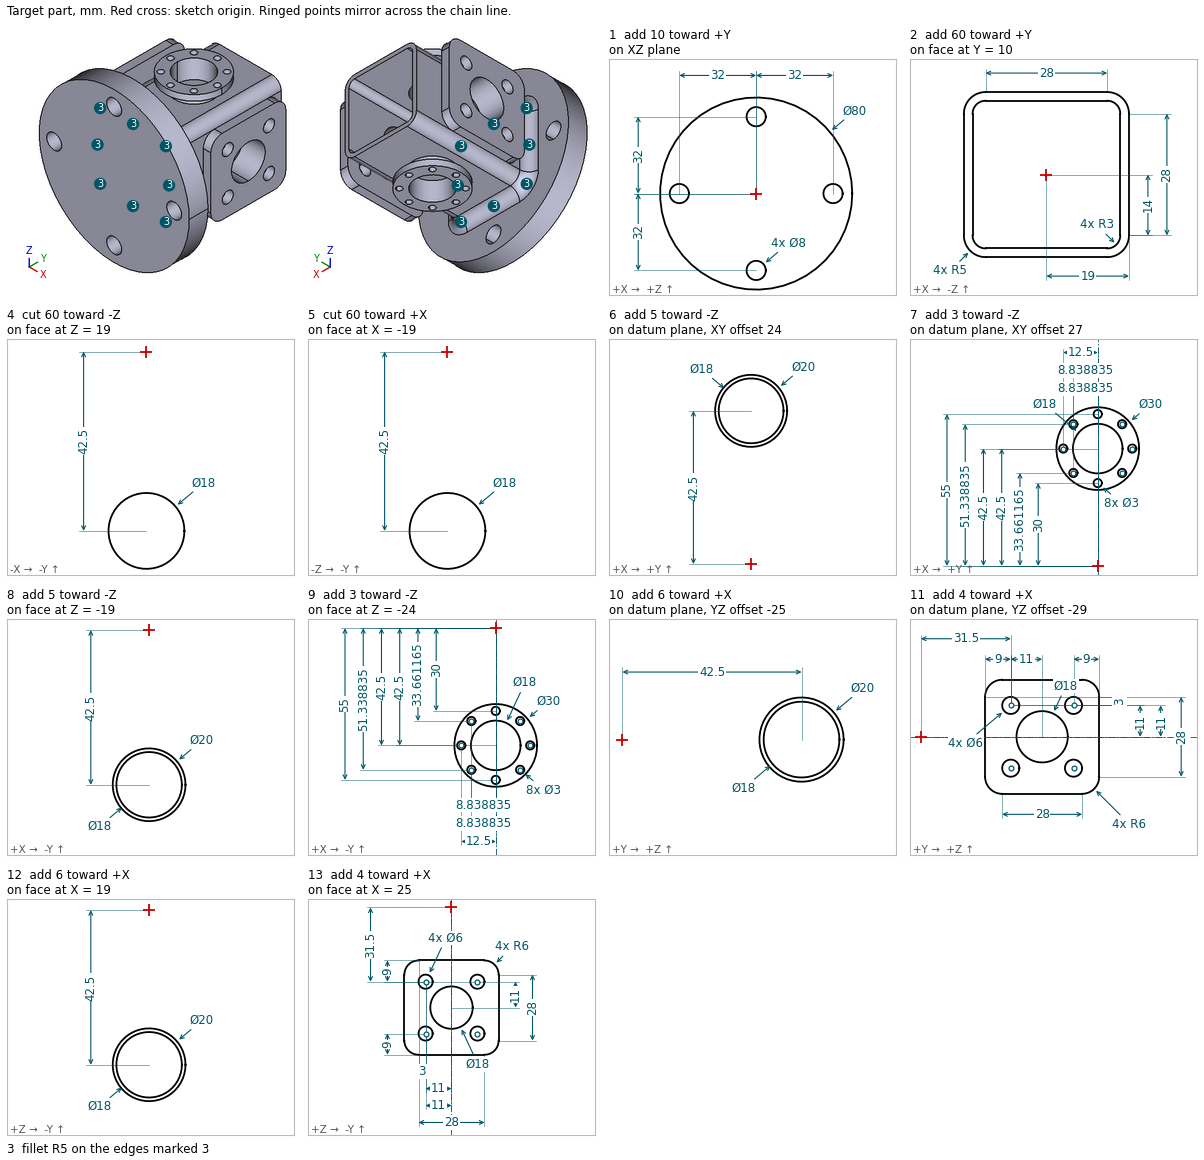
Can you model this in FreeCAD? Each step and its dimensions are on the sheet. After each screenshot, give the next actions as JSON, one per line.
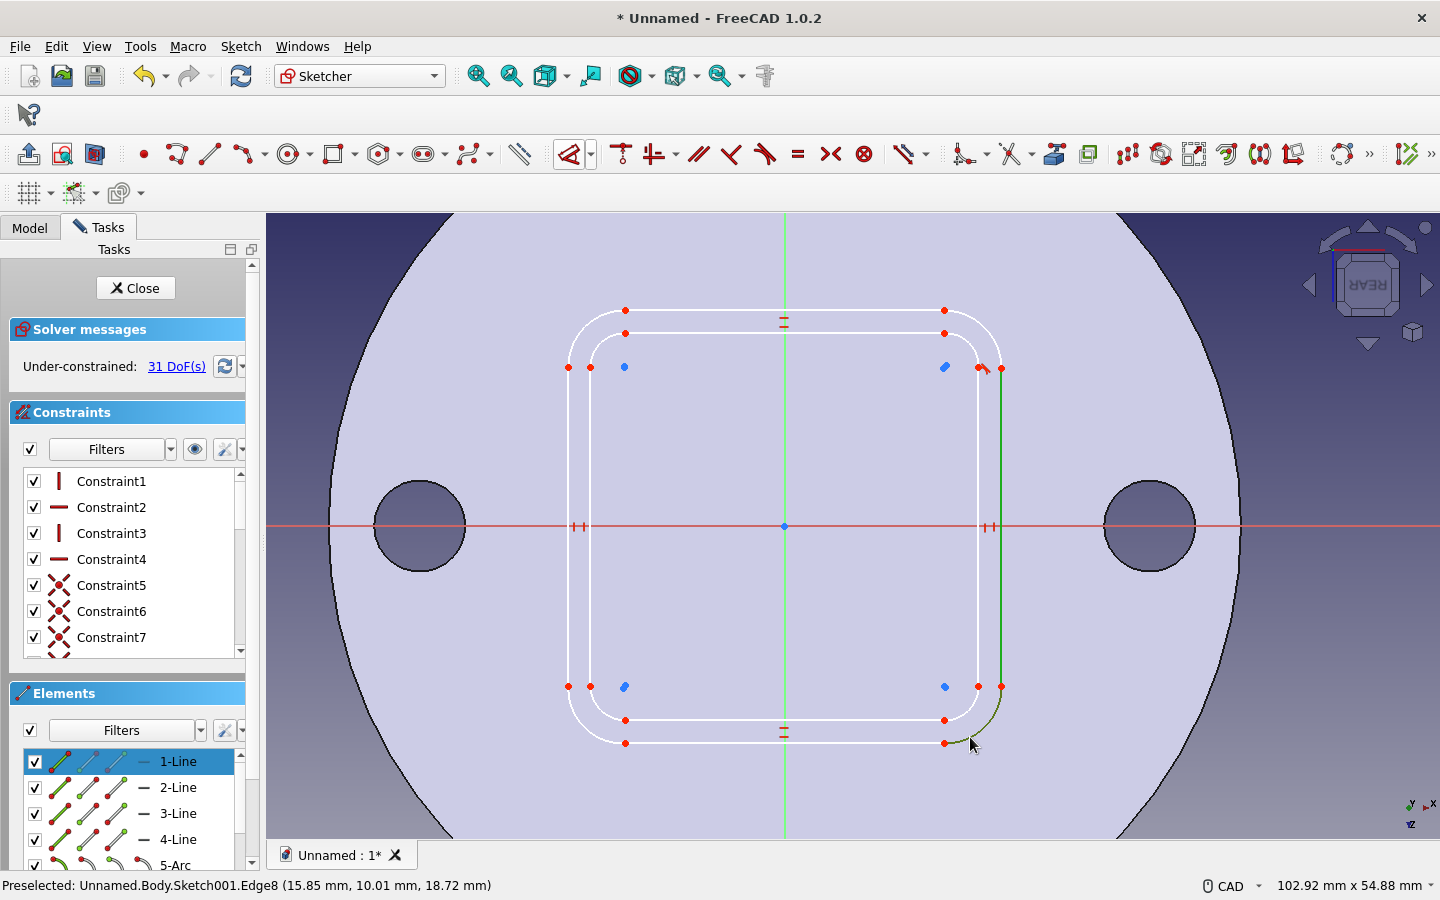
{"action": "key", "text": "t"}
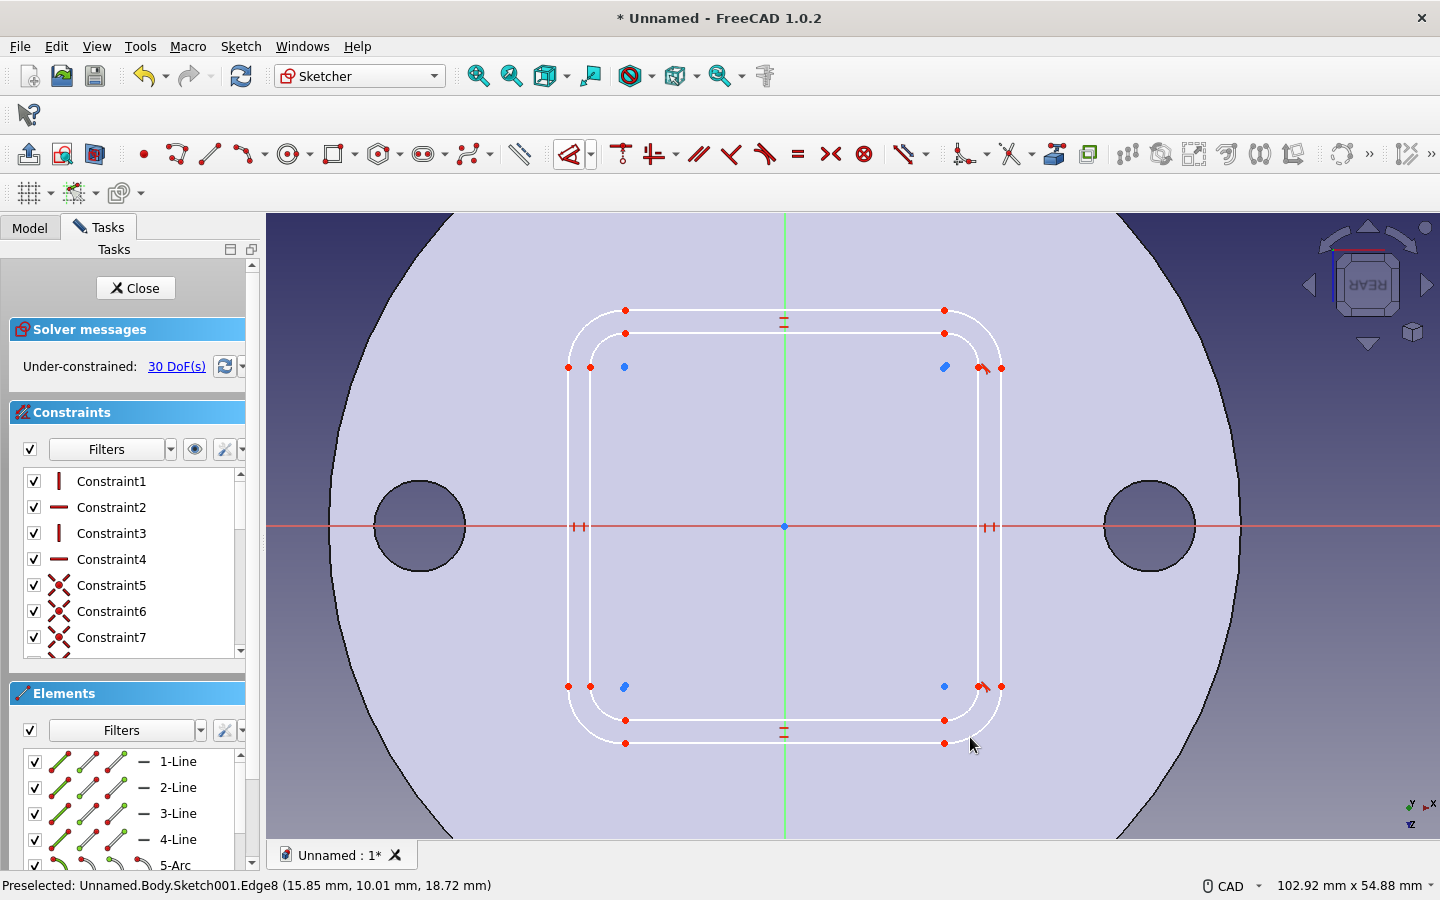
{"action": "left_click", "coordinate": [849, 310]}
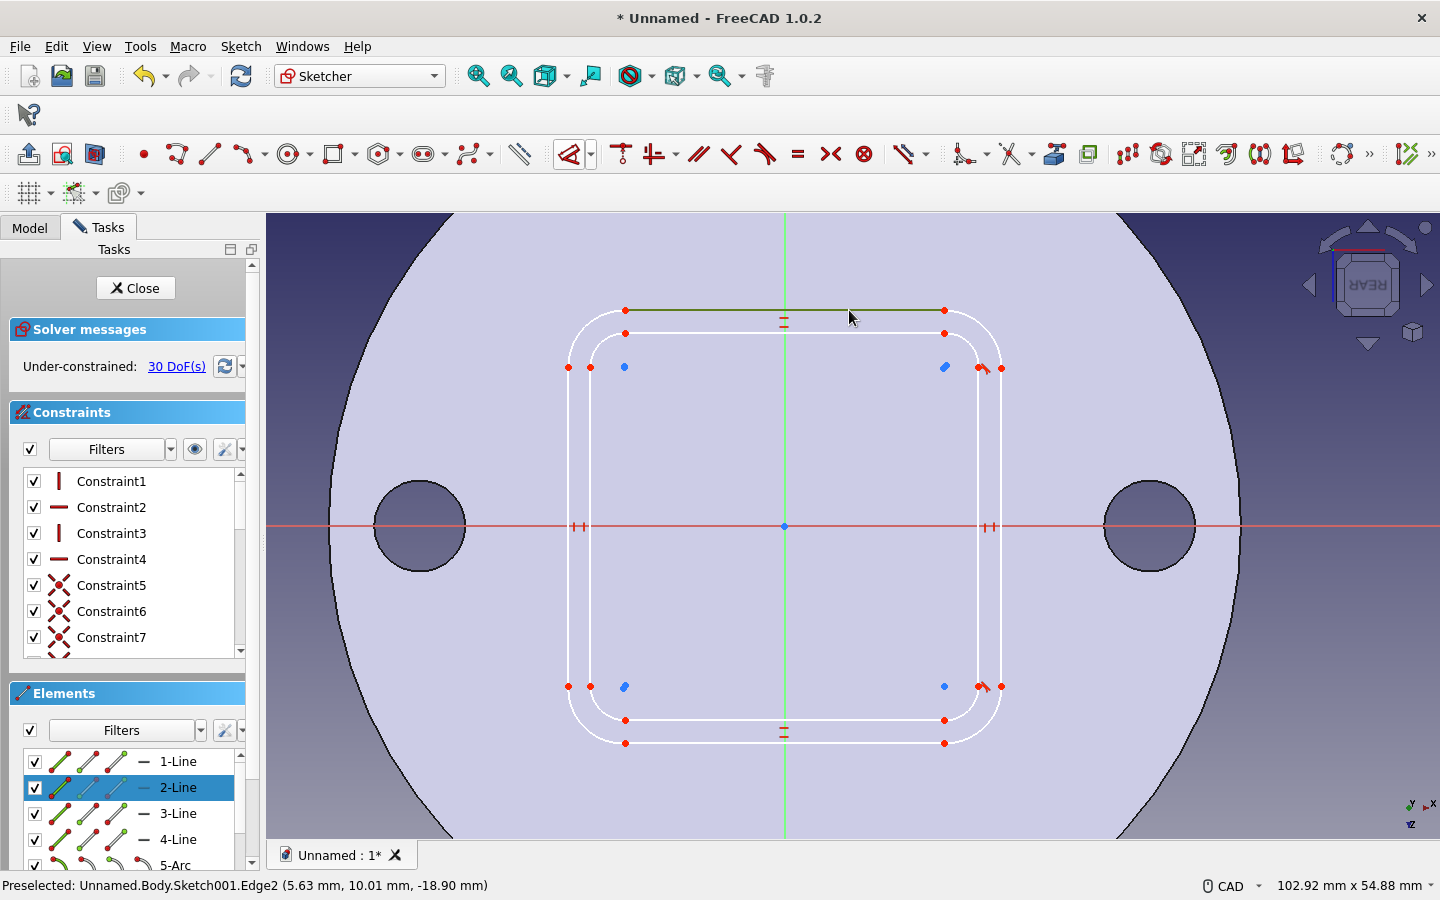
{"action": "left_click", "coordinate": [995, 342]}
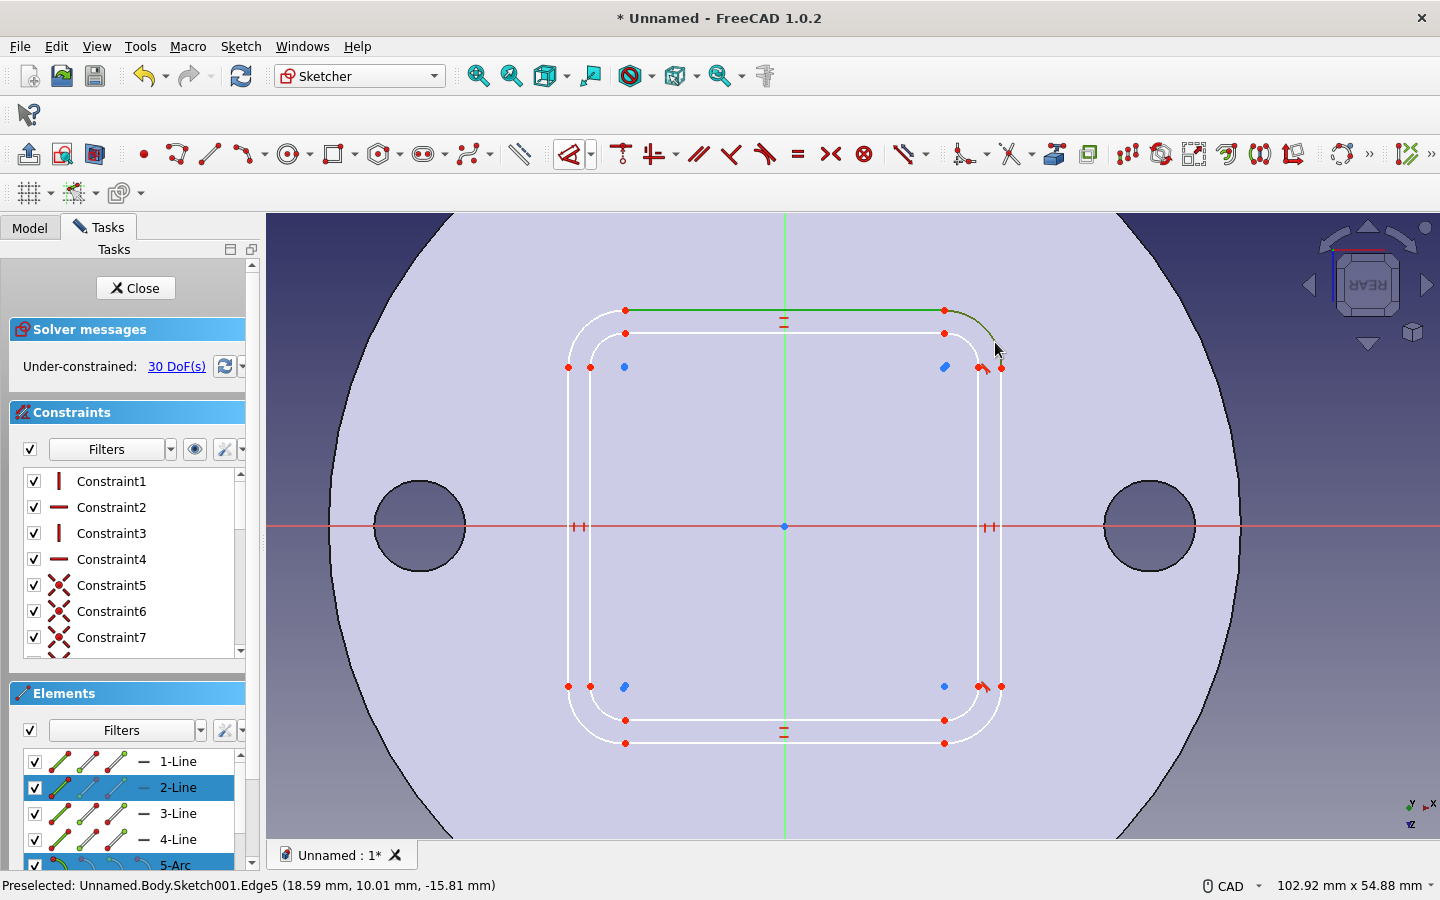
{"action": "key", "text": "t"}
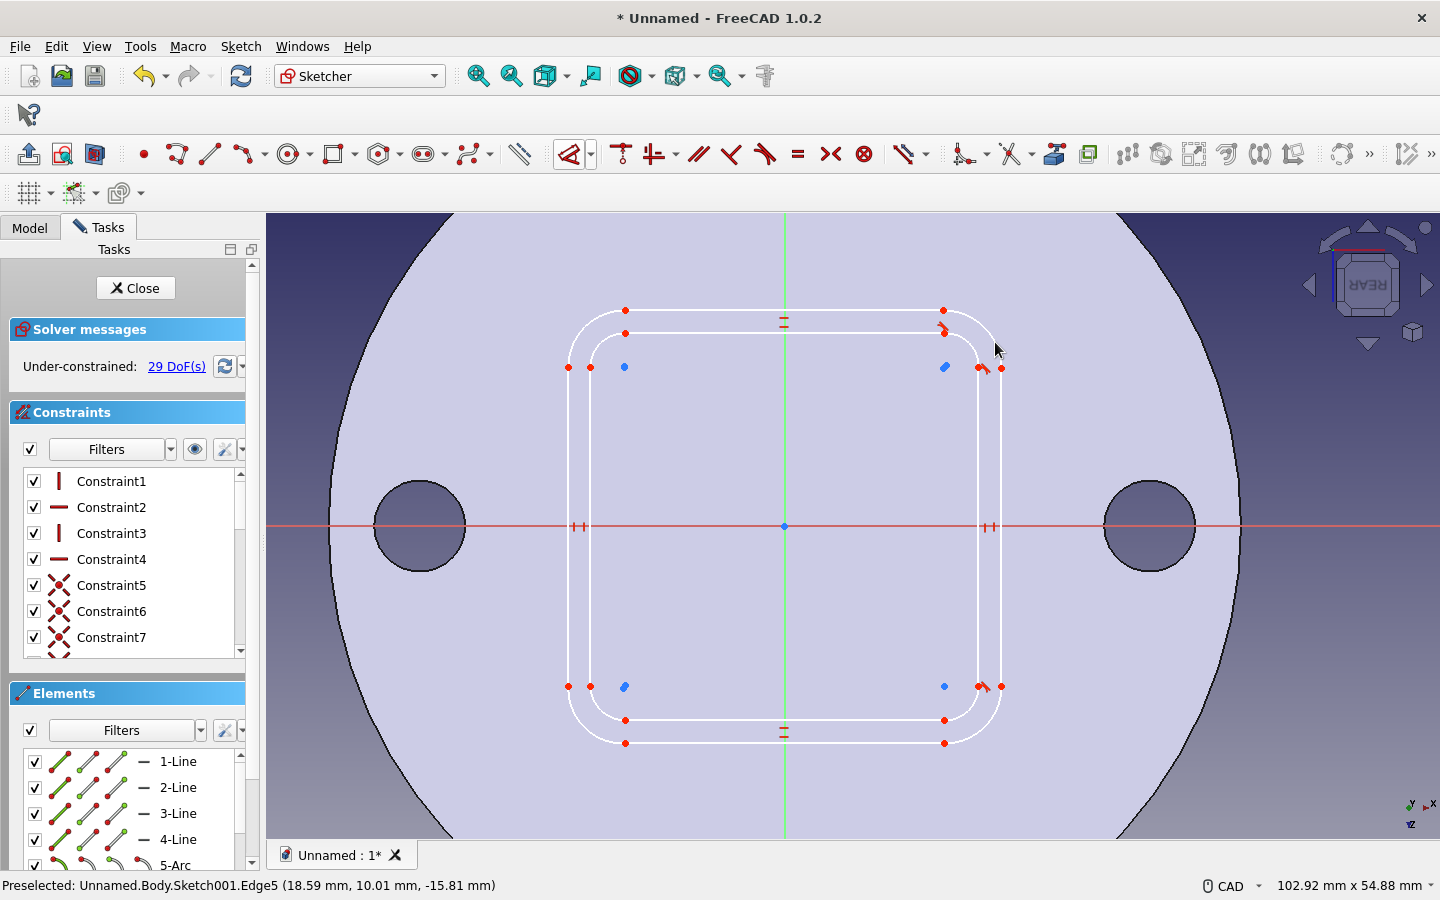
{"action": "left_click", "coordinate": [848, 310]}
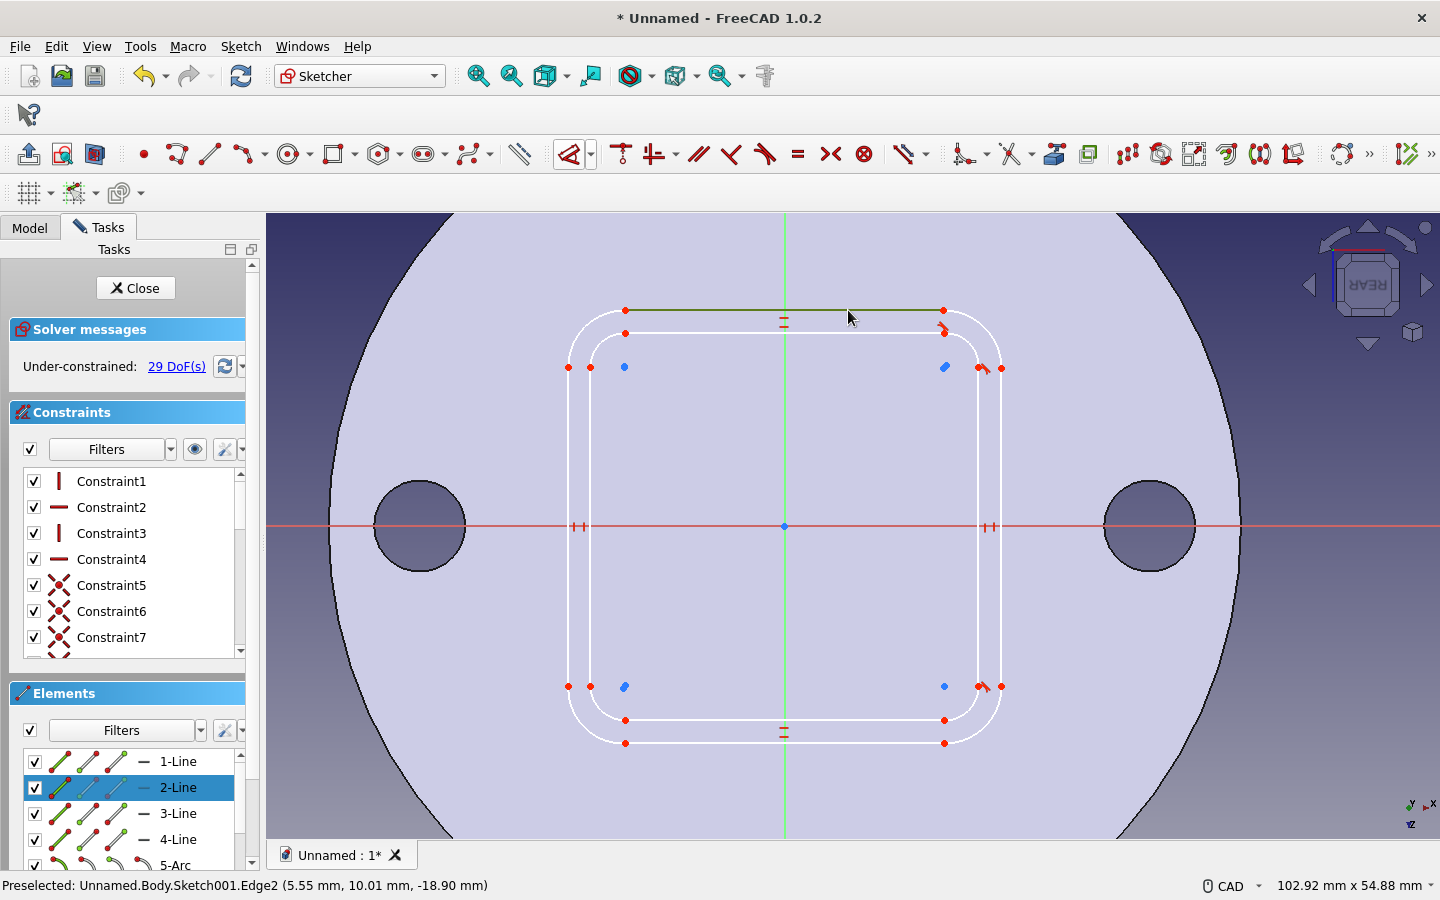
{"action": "left_click", "coordinate": [599, 316]}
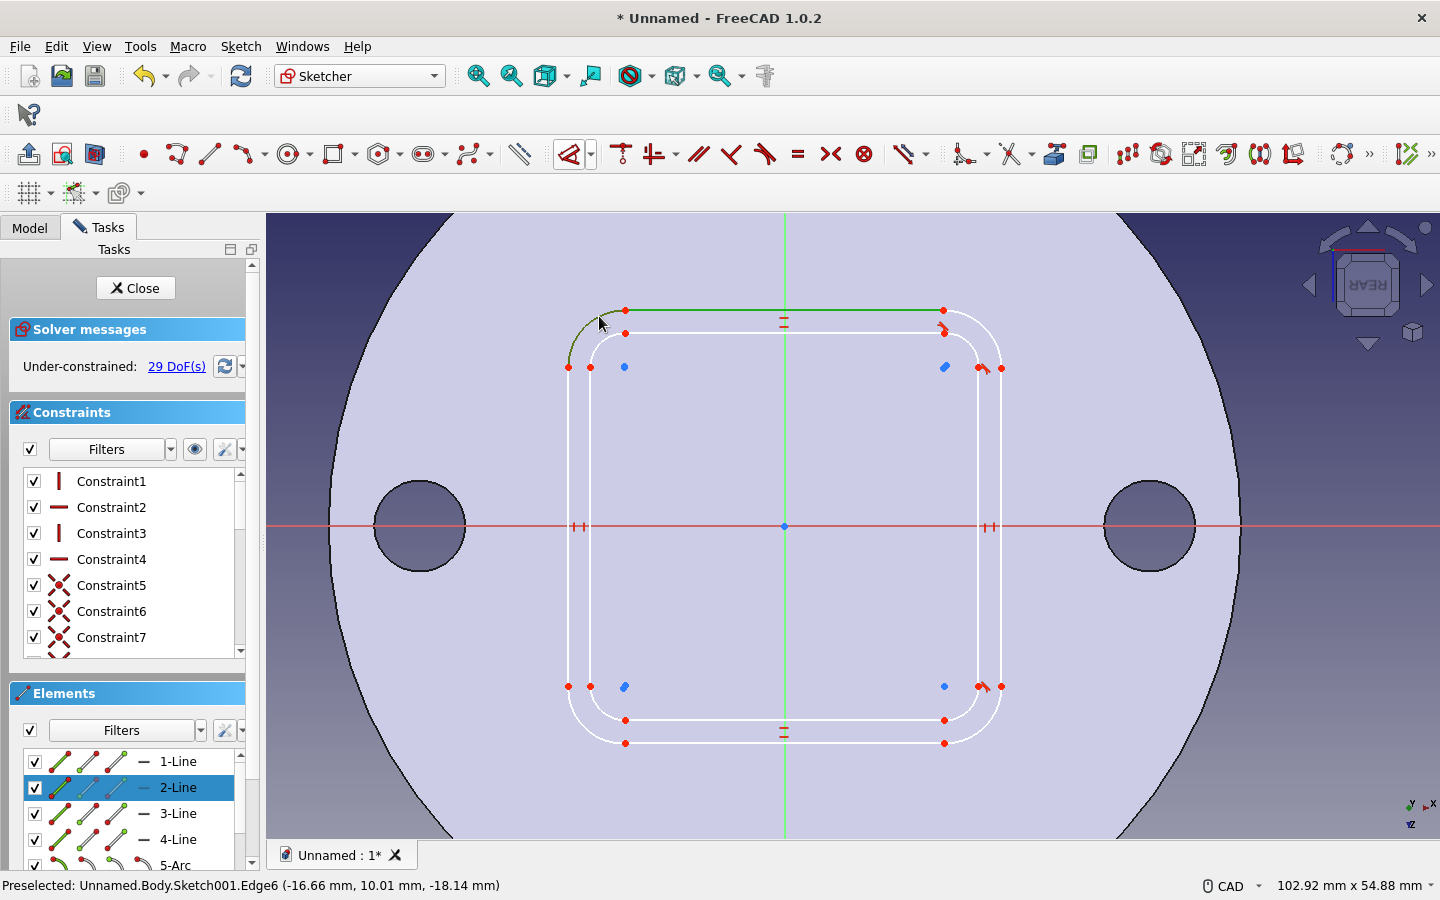
{"action": "left_click", "coordinate": [765, 154]}